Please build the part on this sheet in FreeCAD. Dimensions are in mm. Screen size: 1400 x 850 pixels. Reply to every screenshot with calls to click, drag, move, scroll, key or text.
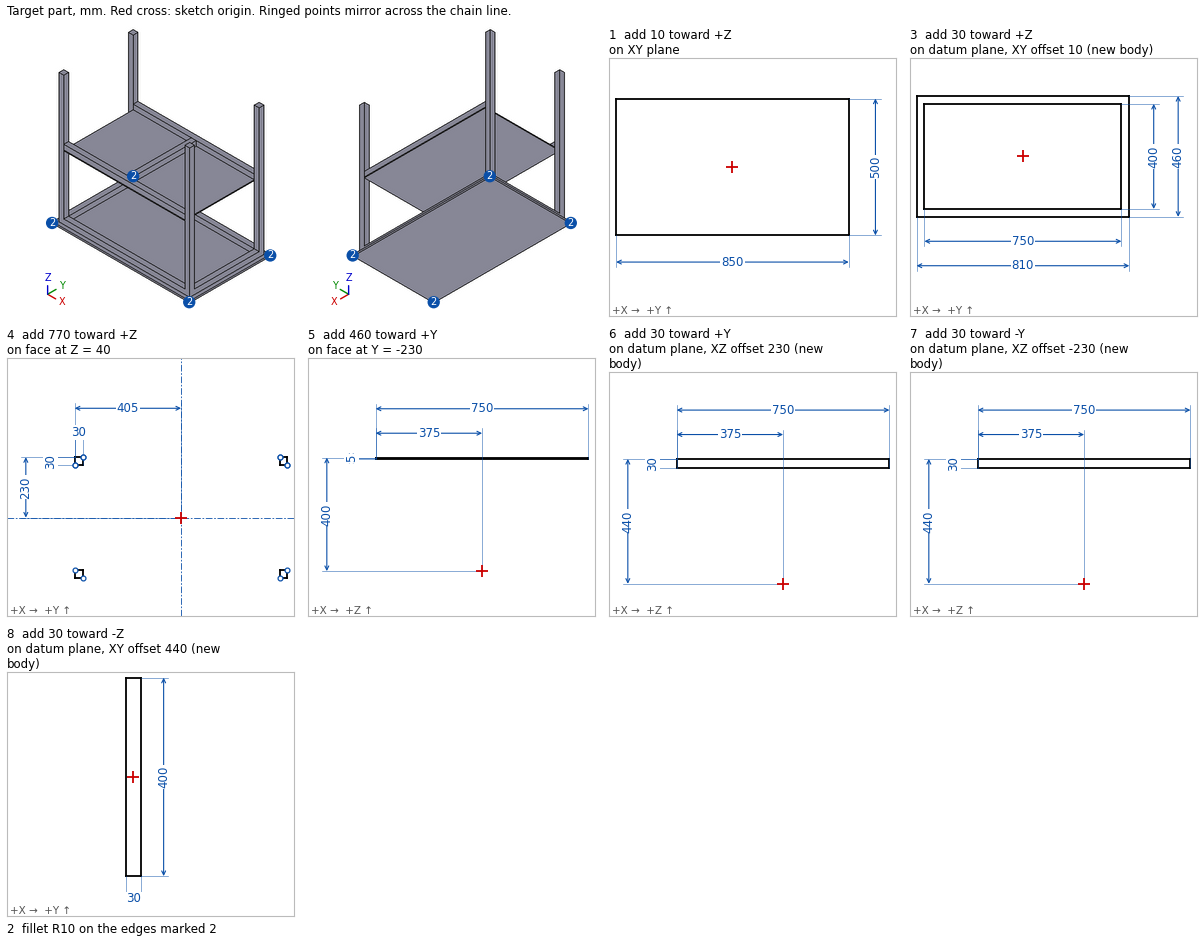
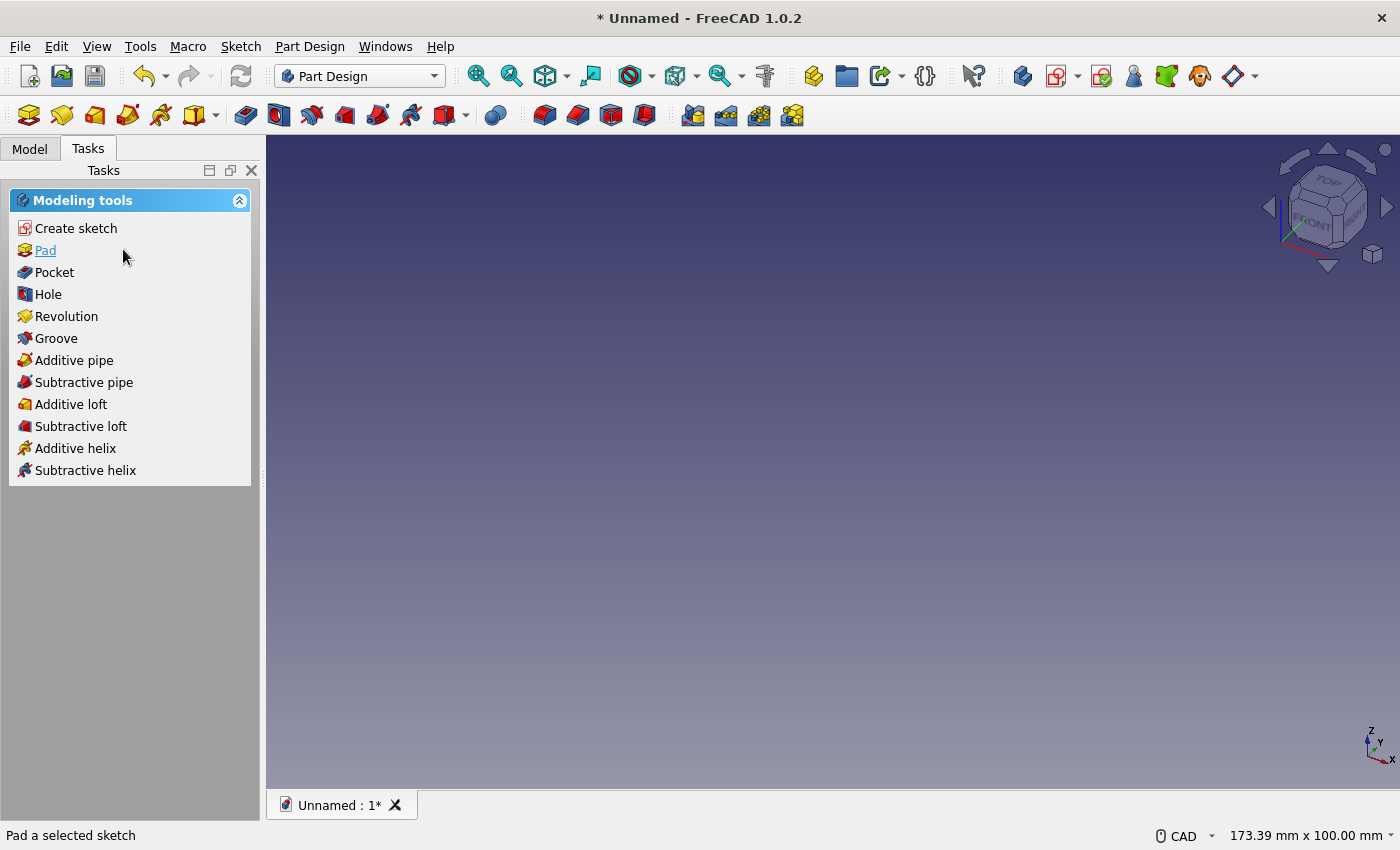
click(29, 116)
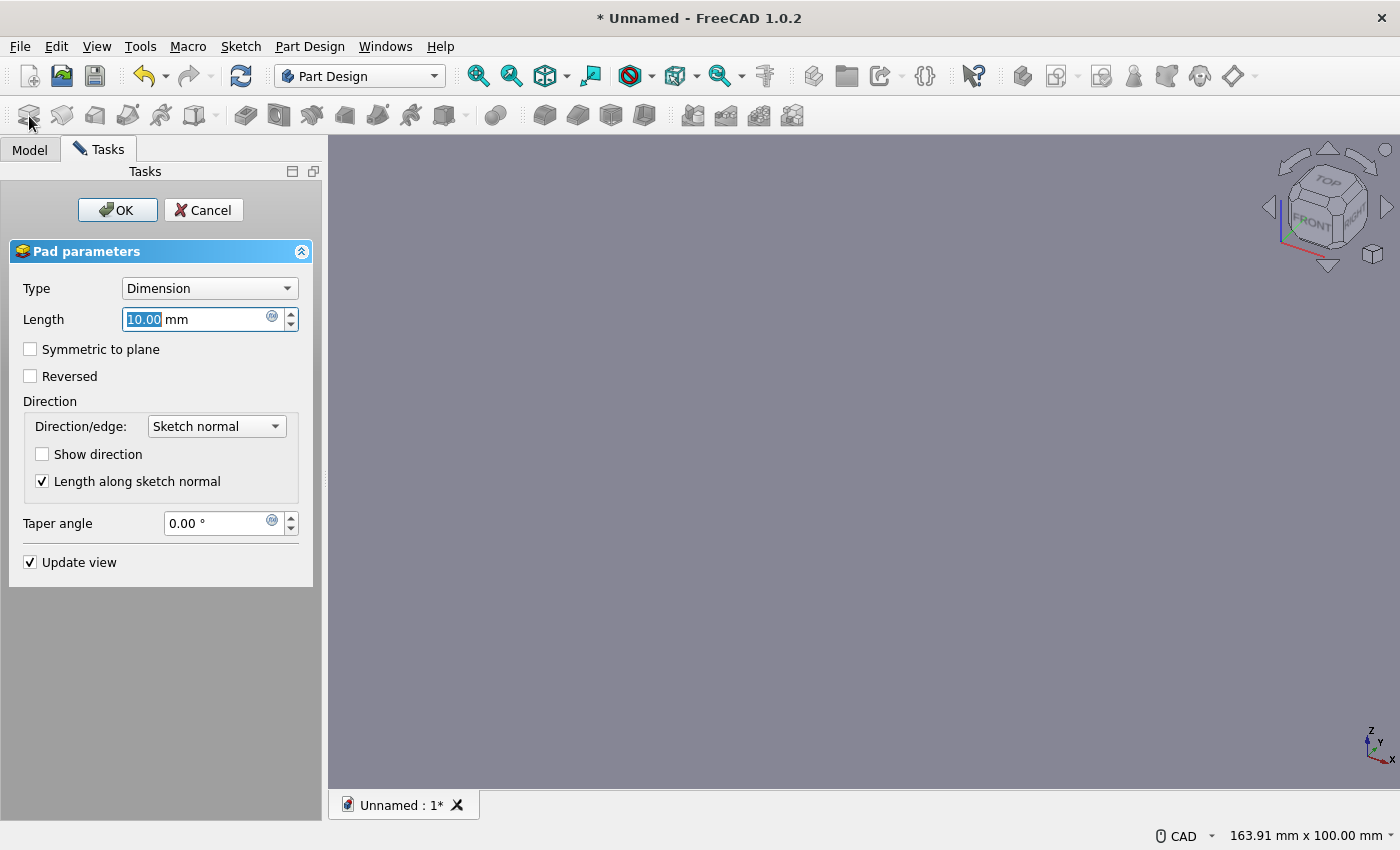
text(10)
key(Tab)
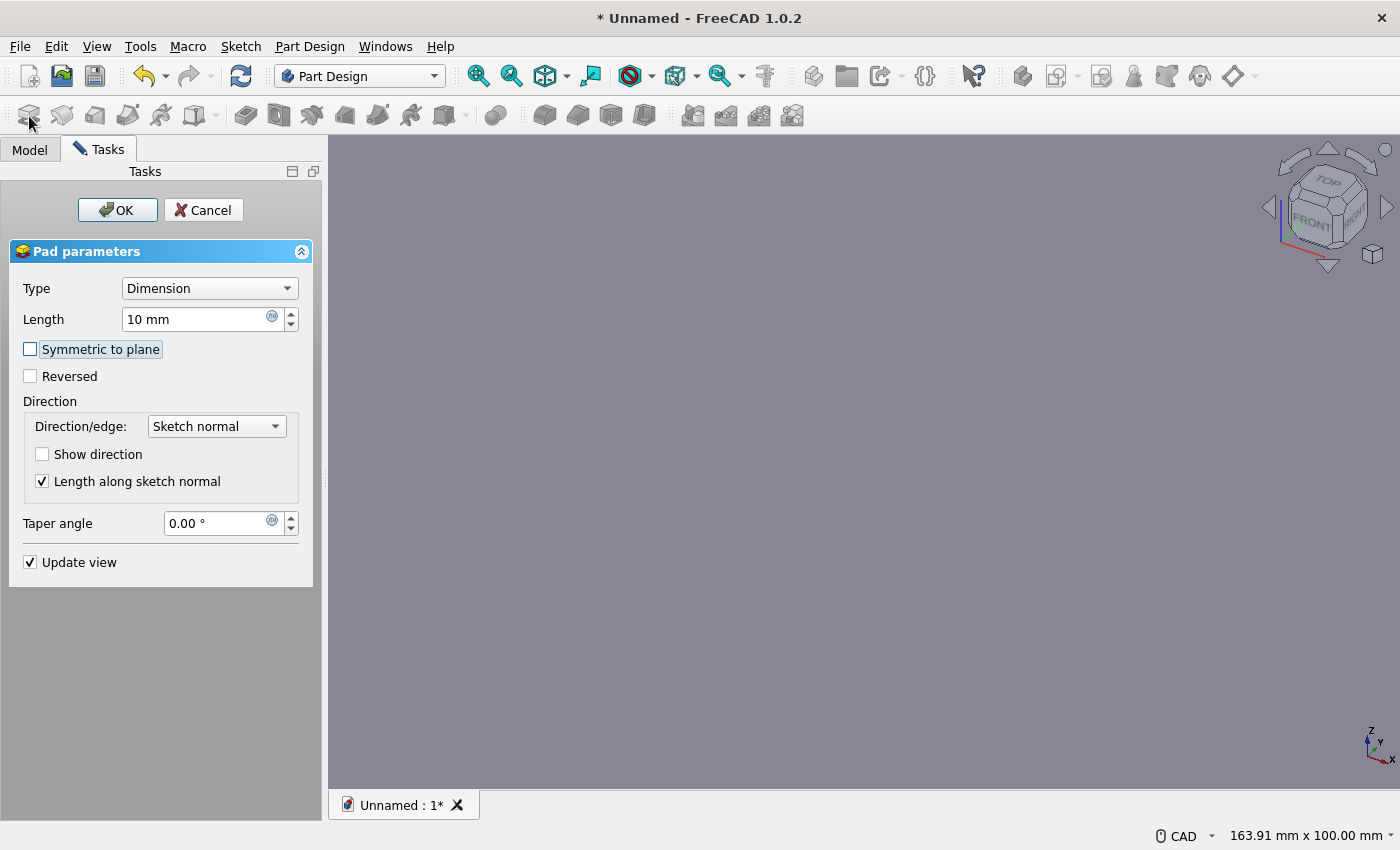
click(118, 210)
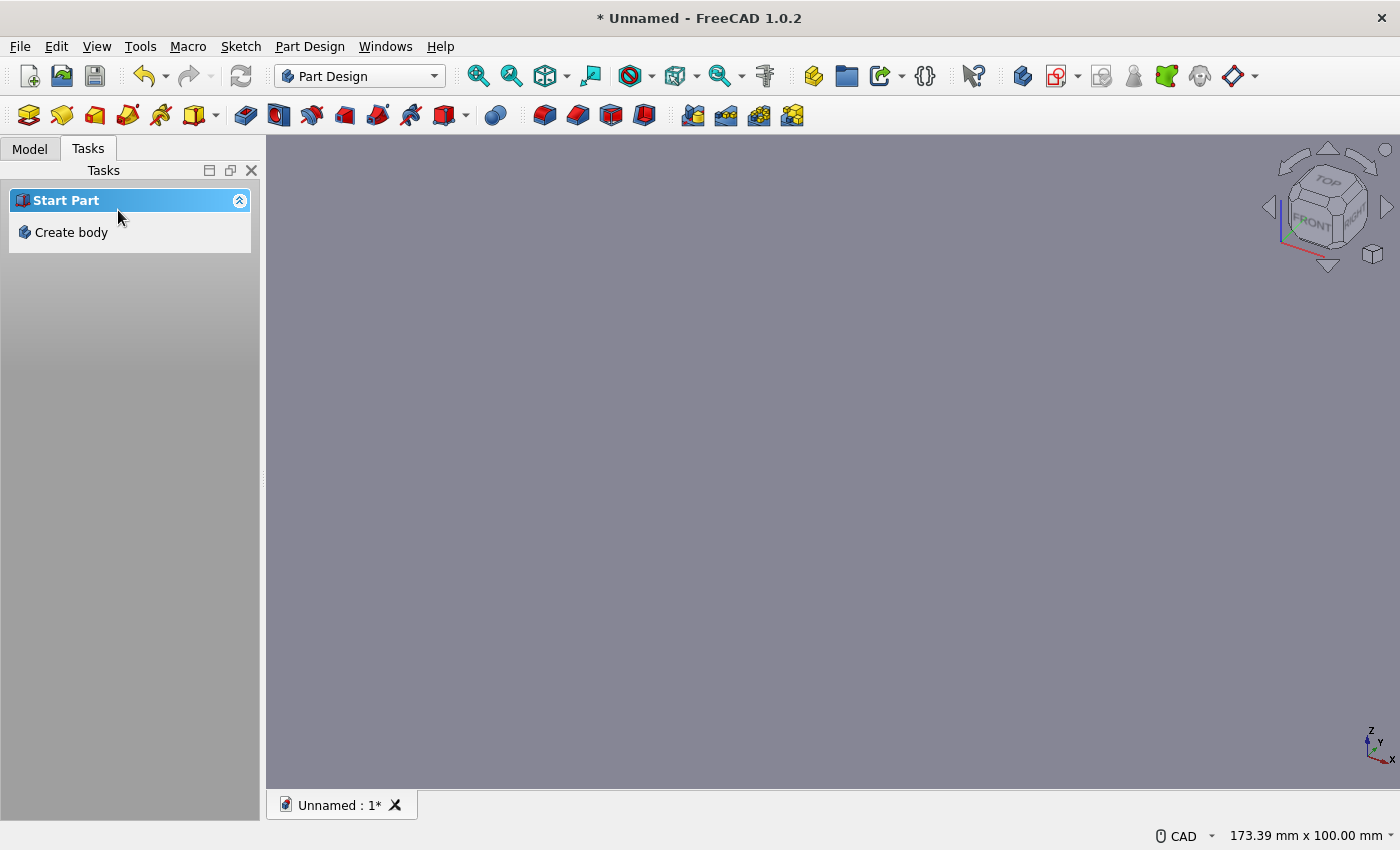
click(479, 76)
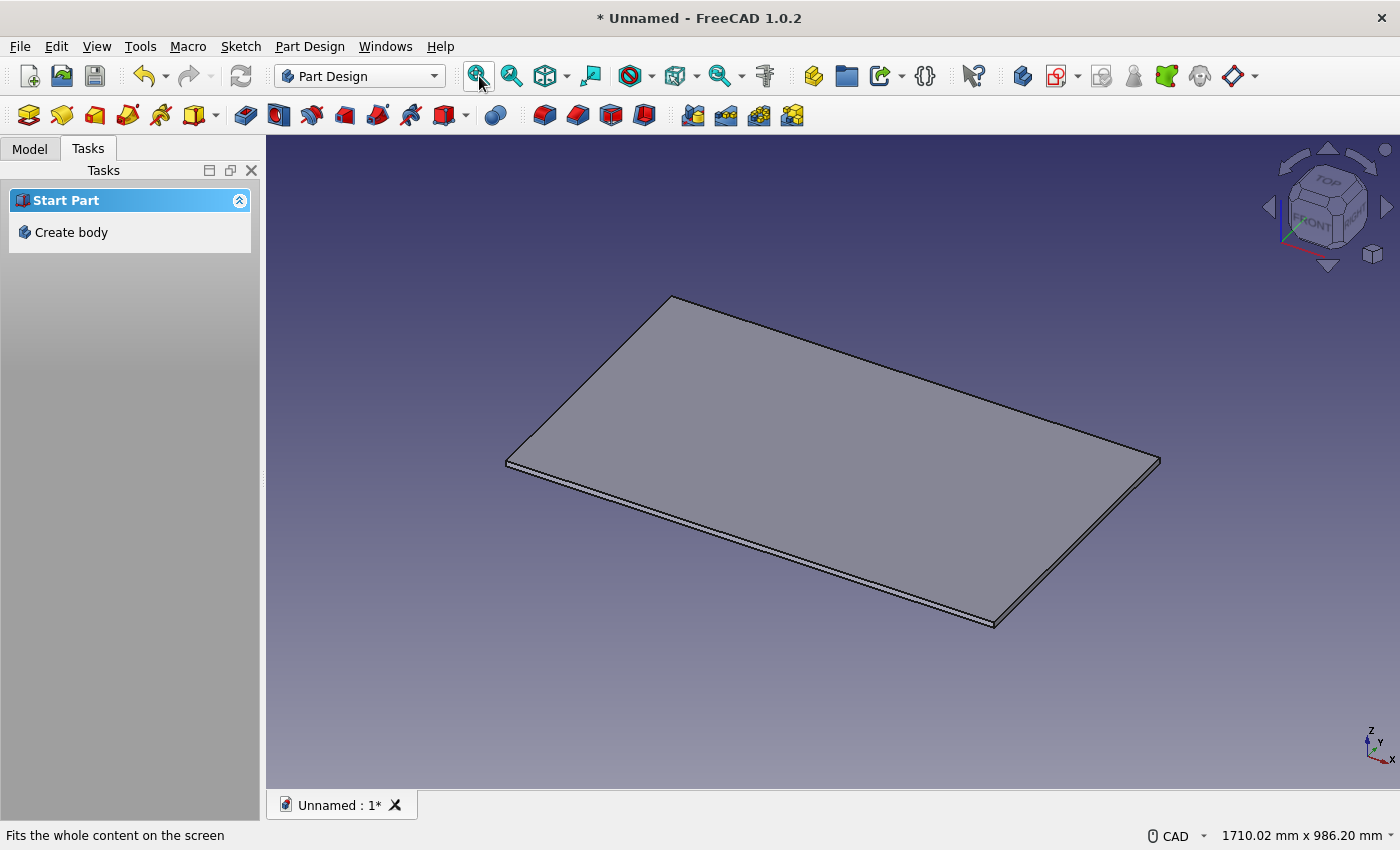
scroll(994, 624, up, 9)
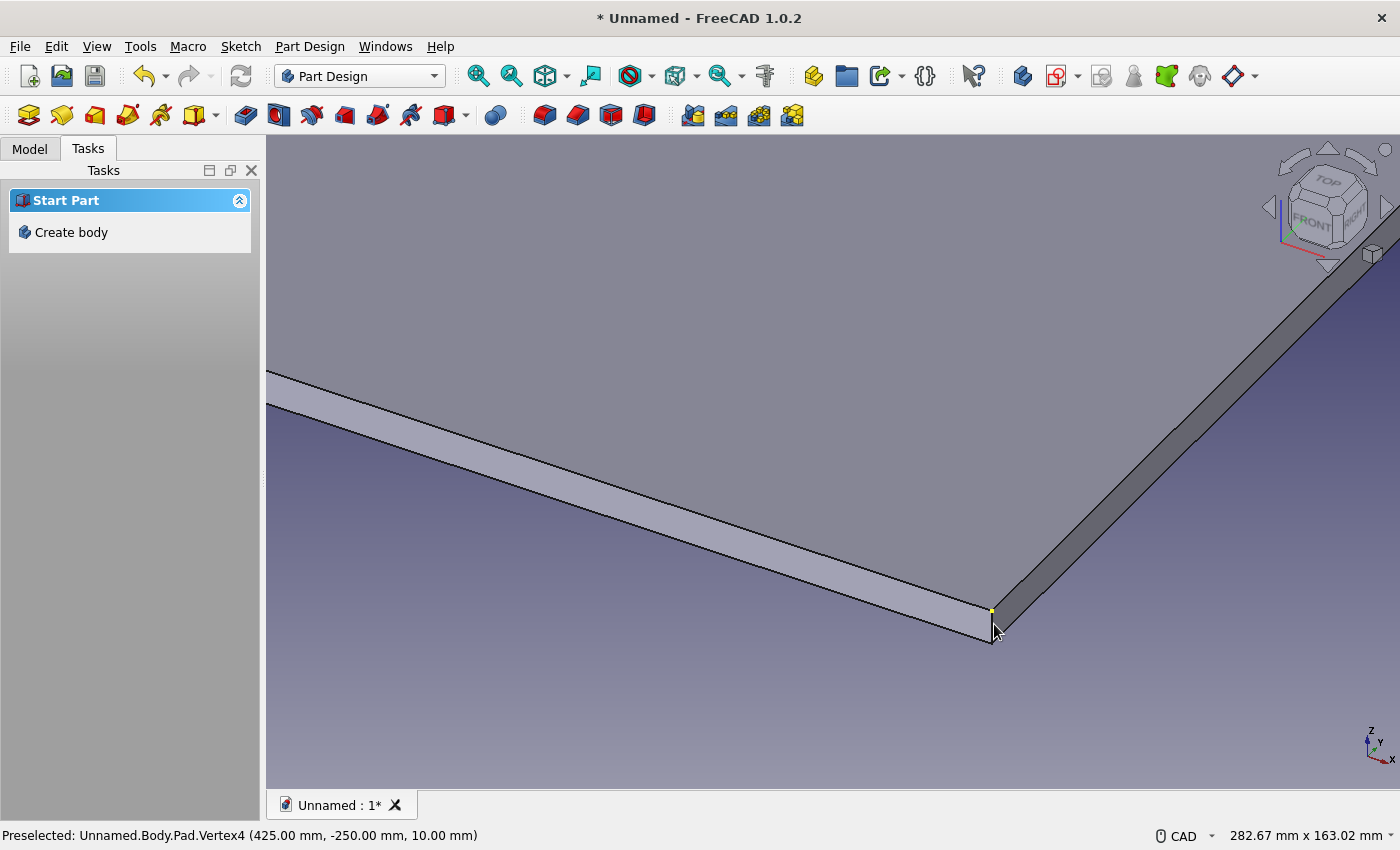
click(992, 626)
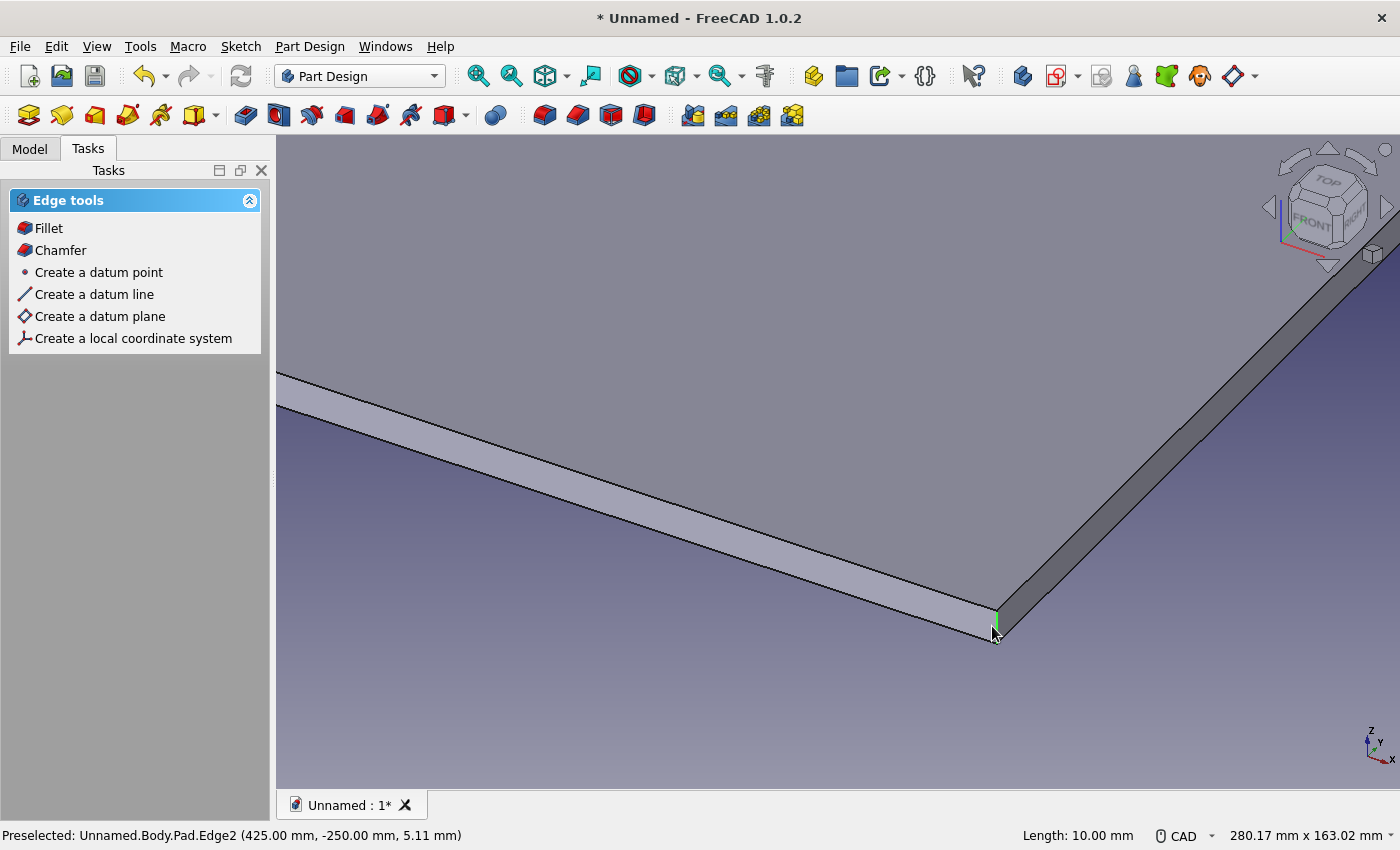
click(479, 76)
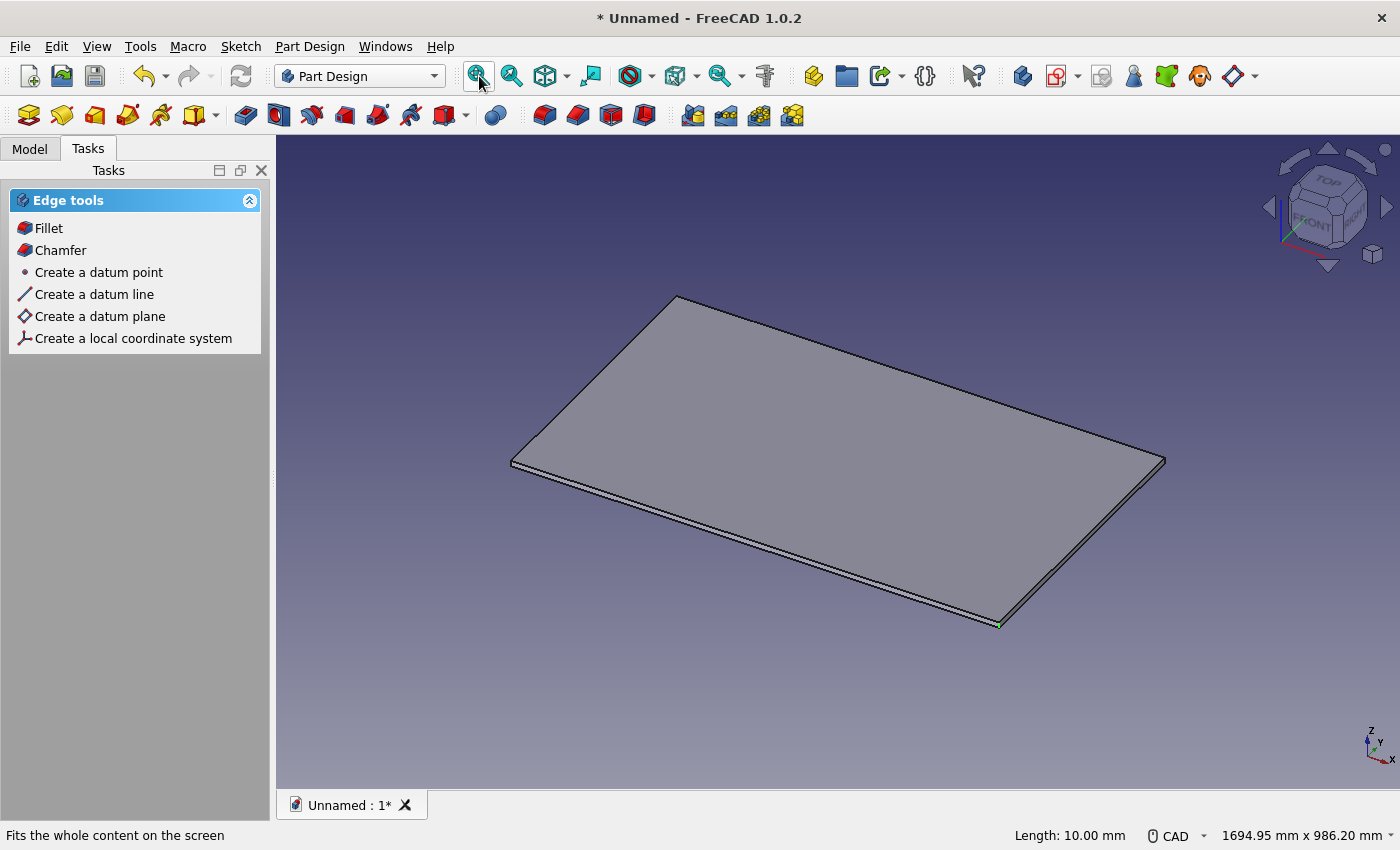
key(0)